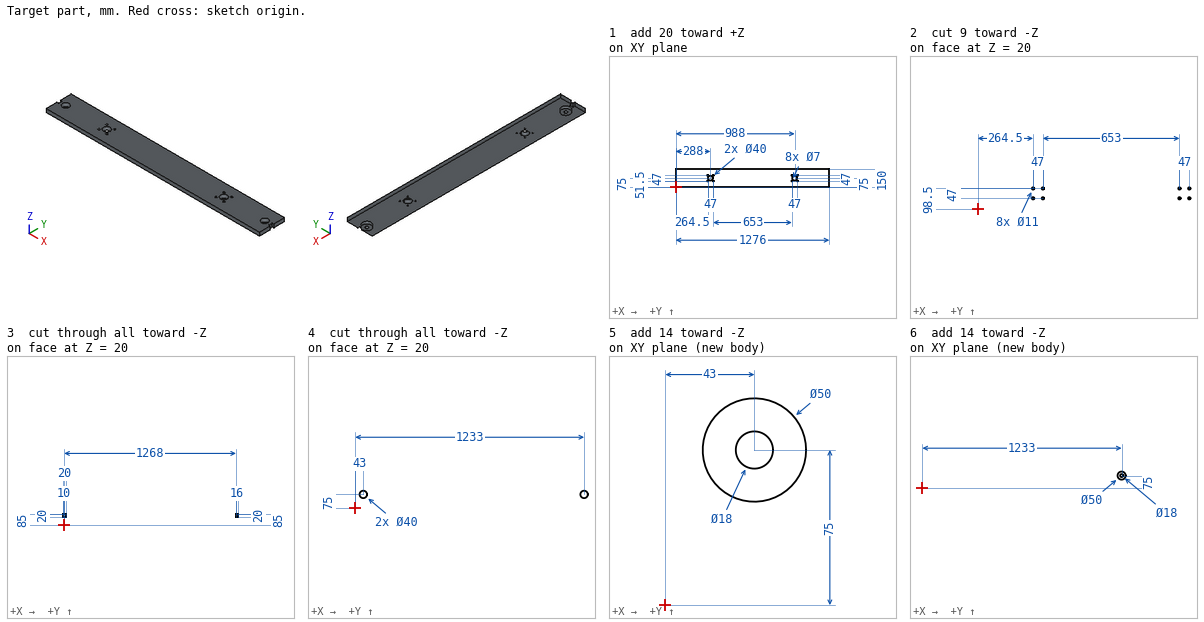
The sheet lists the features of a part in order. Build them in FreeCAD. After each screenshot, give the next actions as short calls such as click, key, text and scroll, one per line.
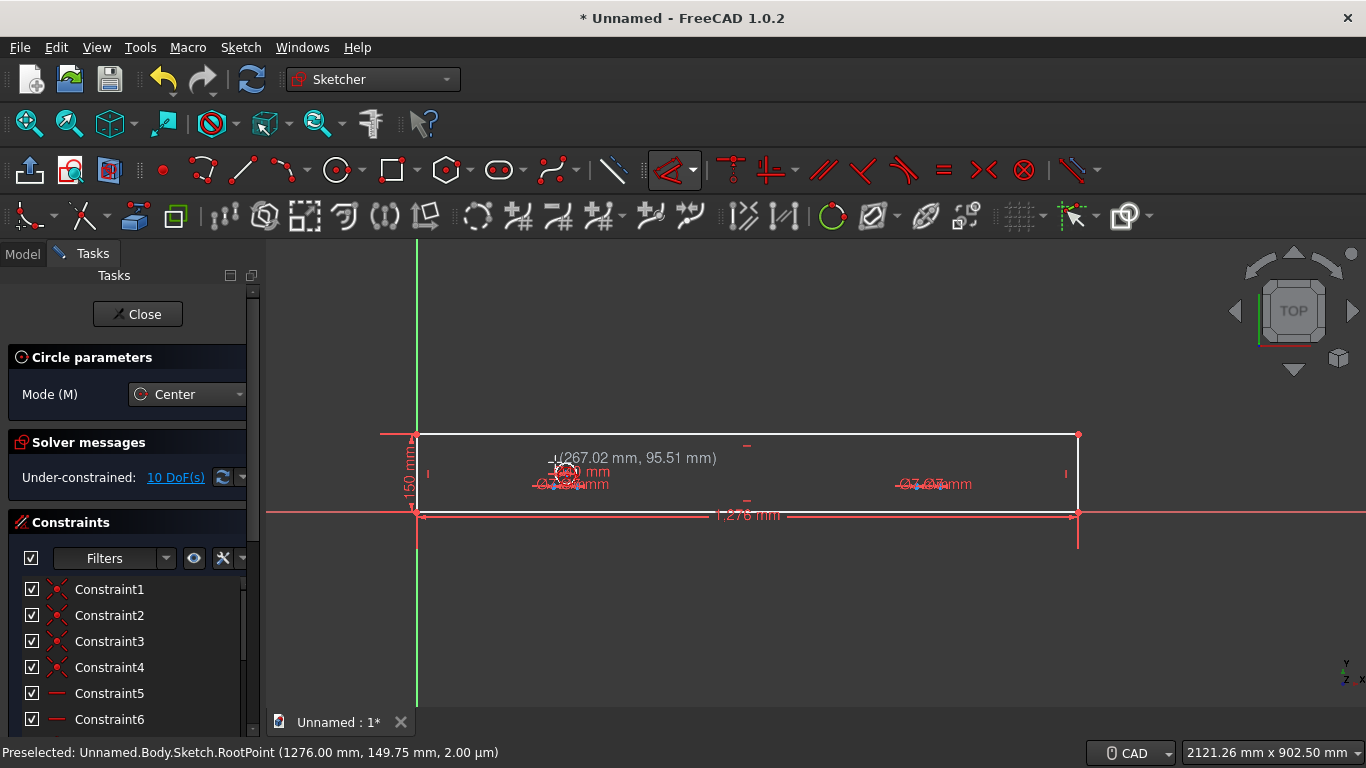
scroll(554, 461, up, 5)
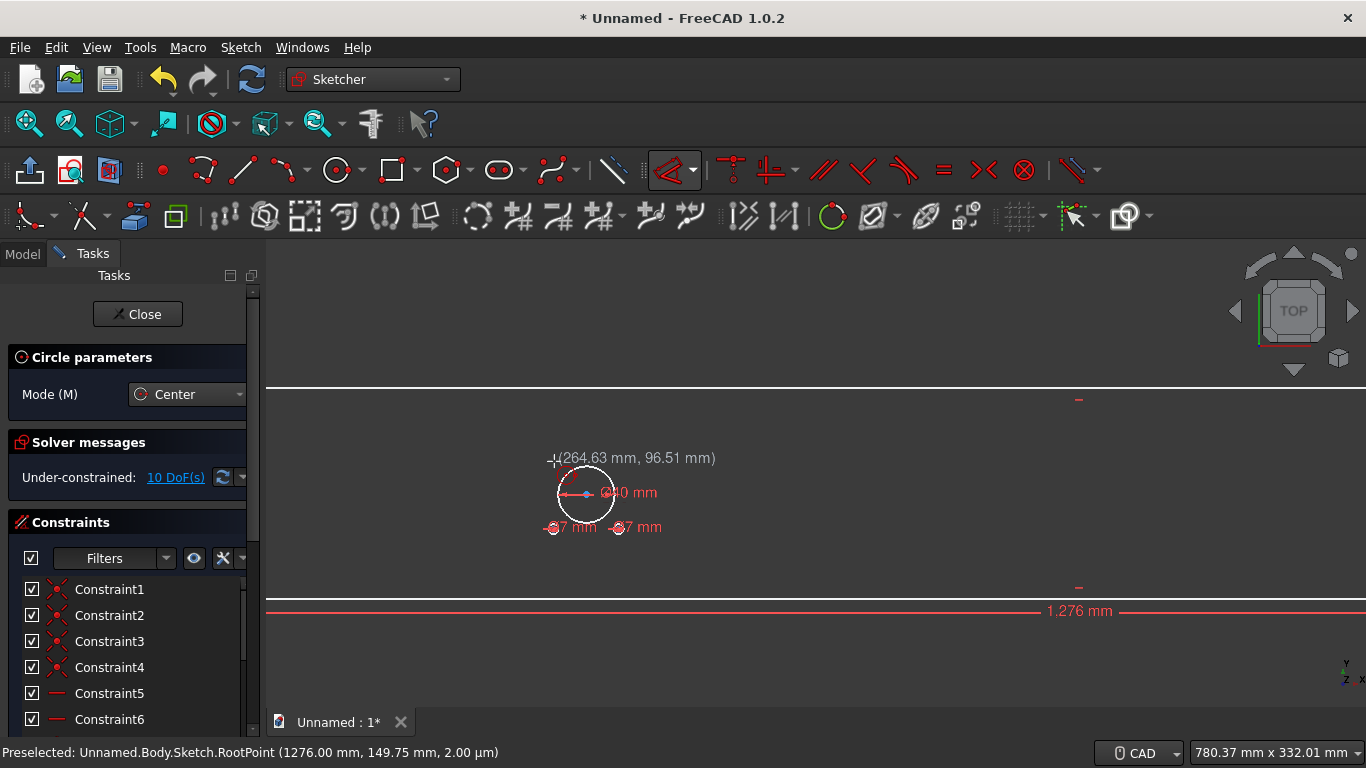
click(553, 460)
move(557, 457)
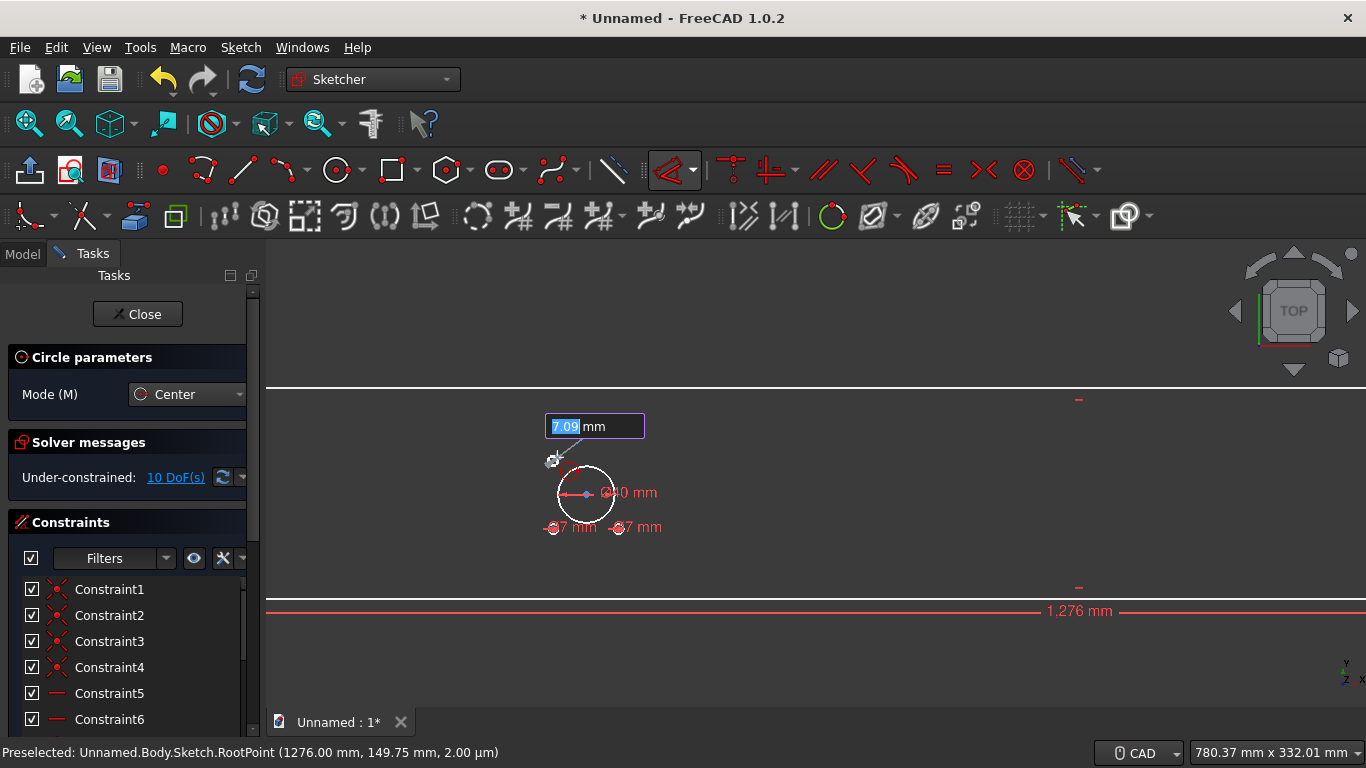
text(7)
key(Return)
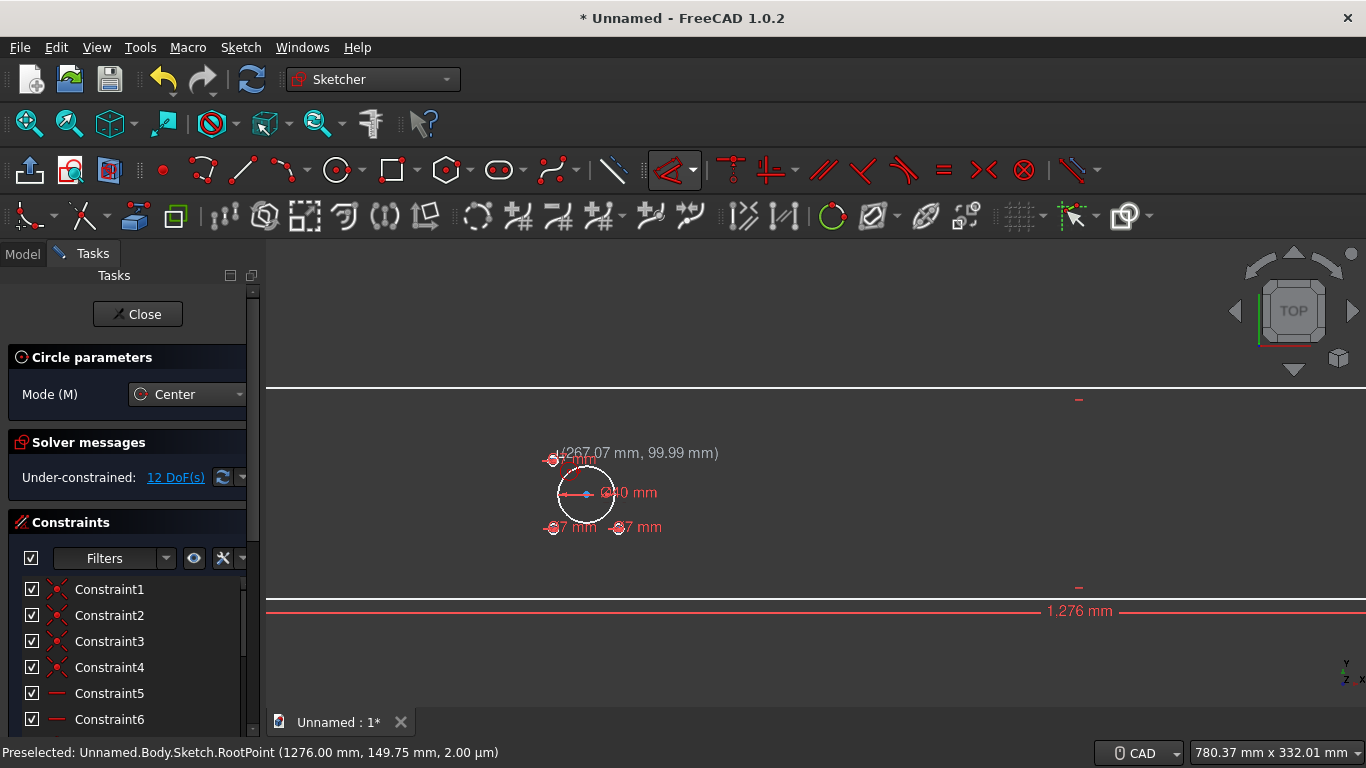
scroll(620, 460, up, 8)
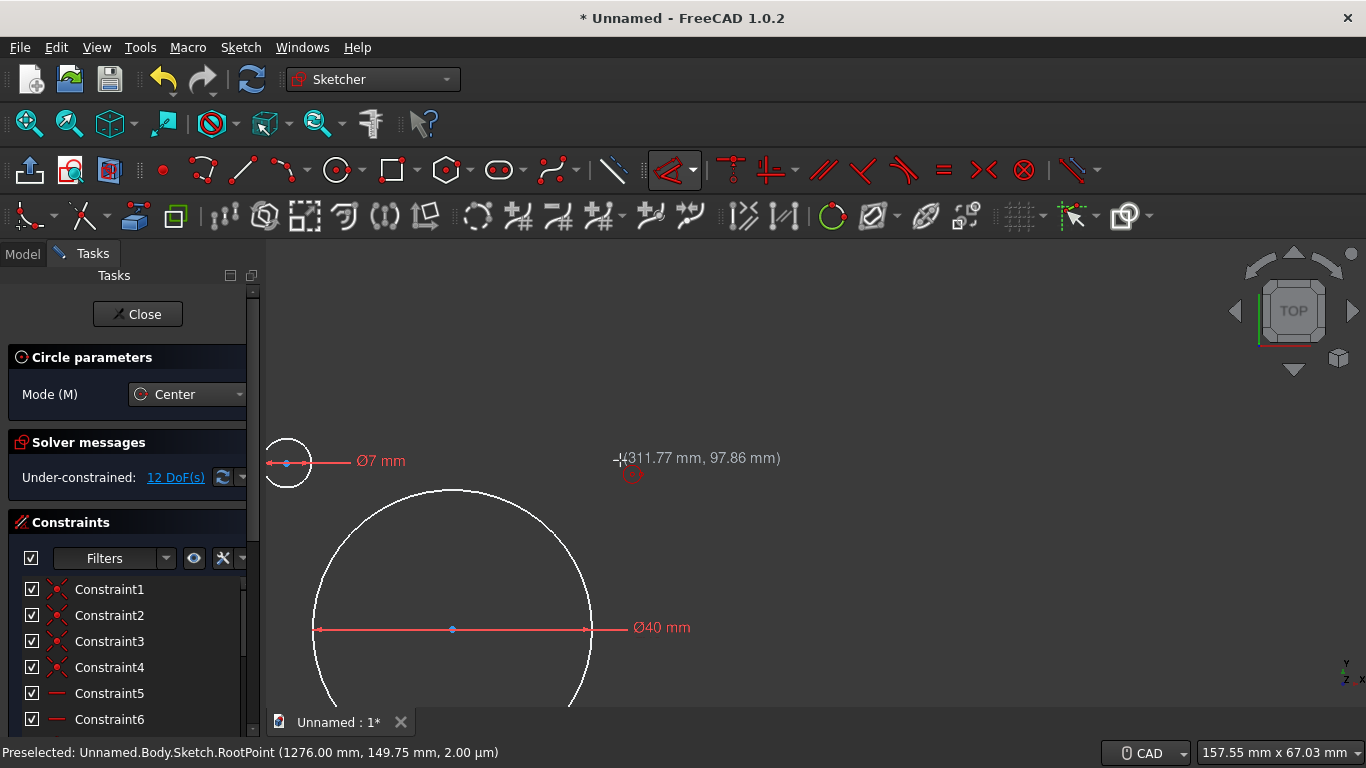
scroll(575, 461, down, 13)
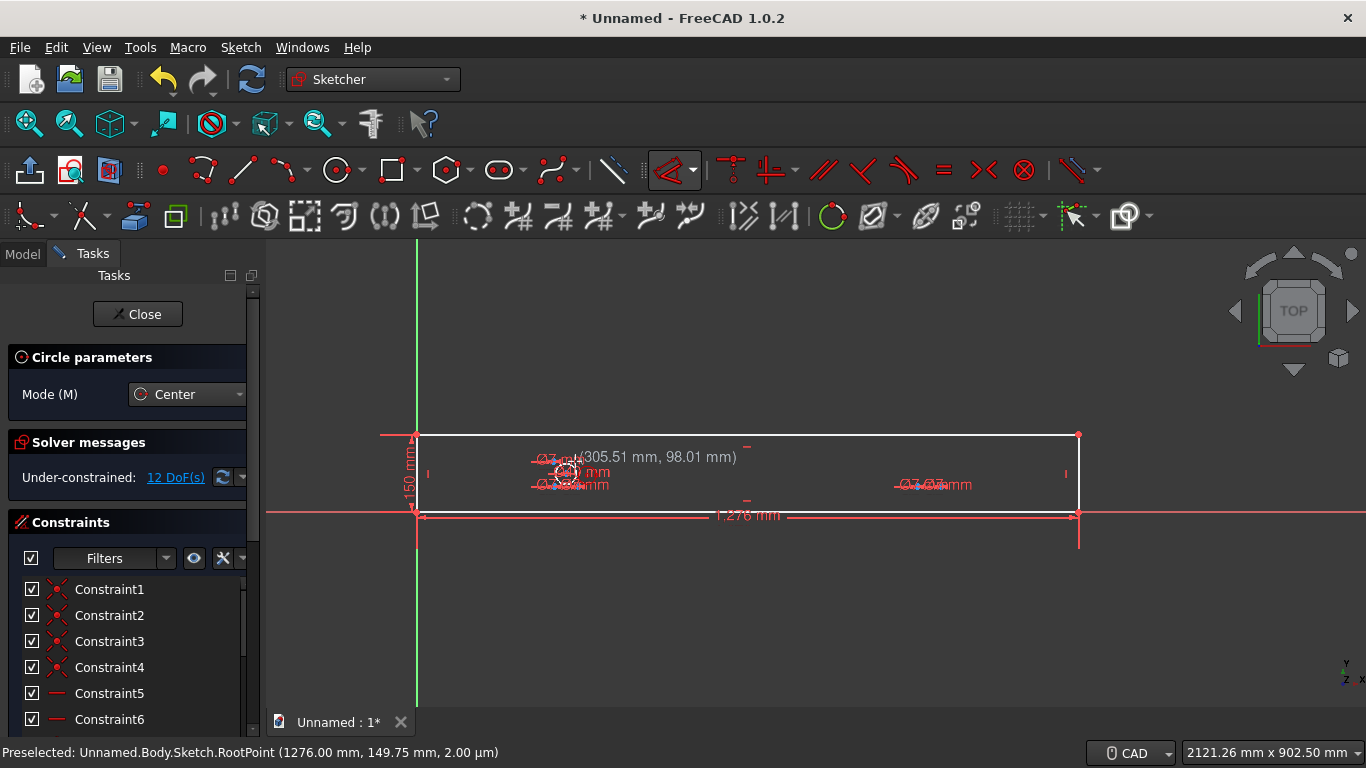
scroll(578, 461, up, 5)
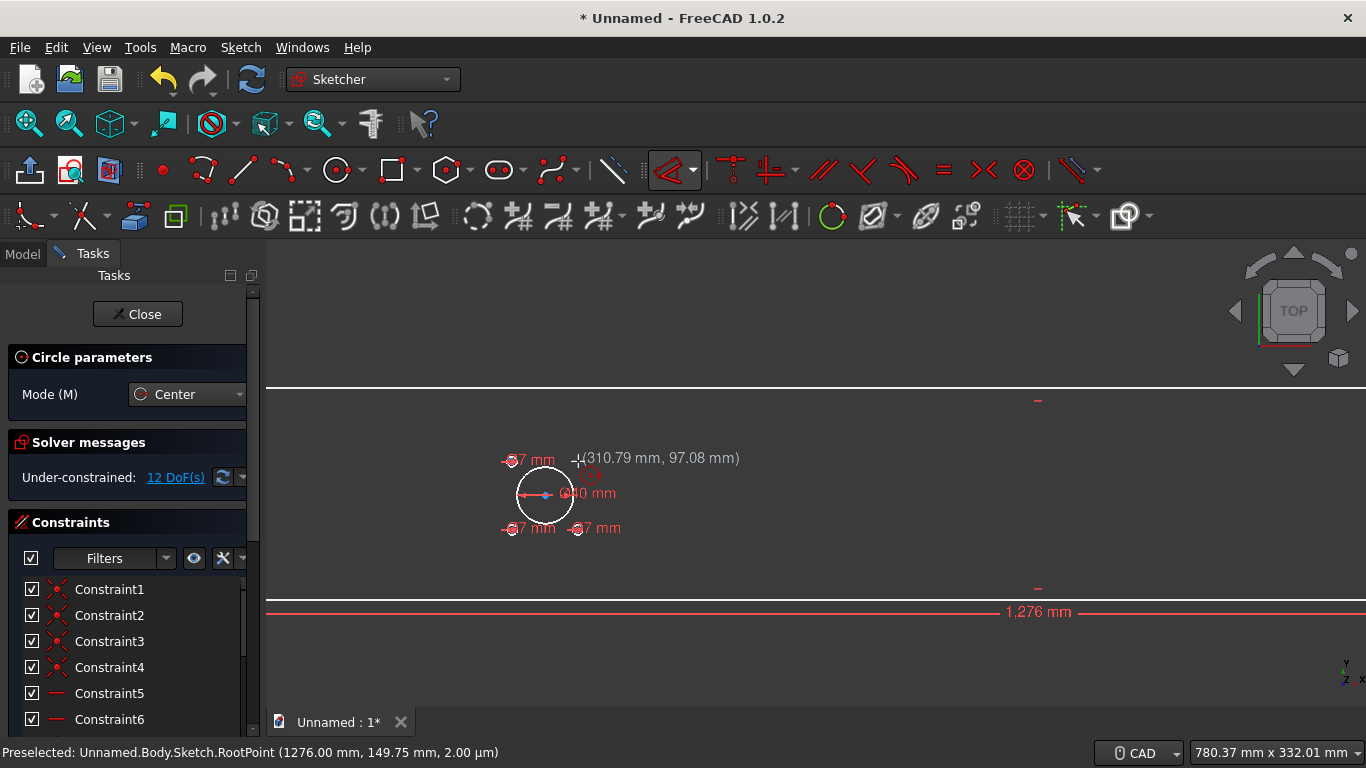
click(579, 461)
move(582, 457)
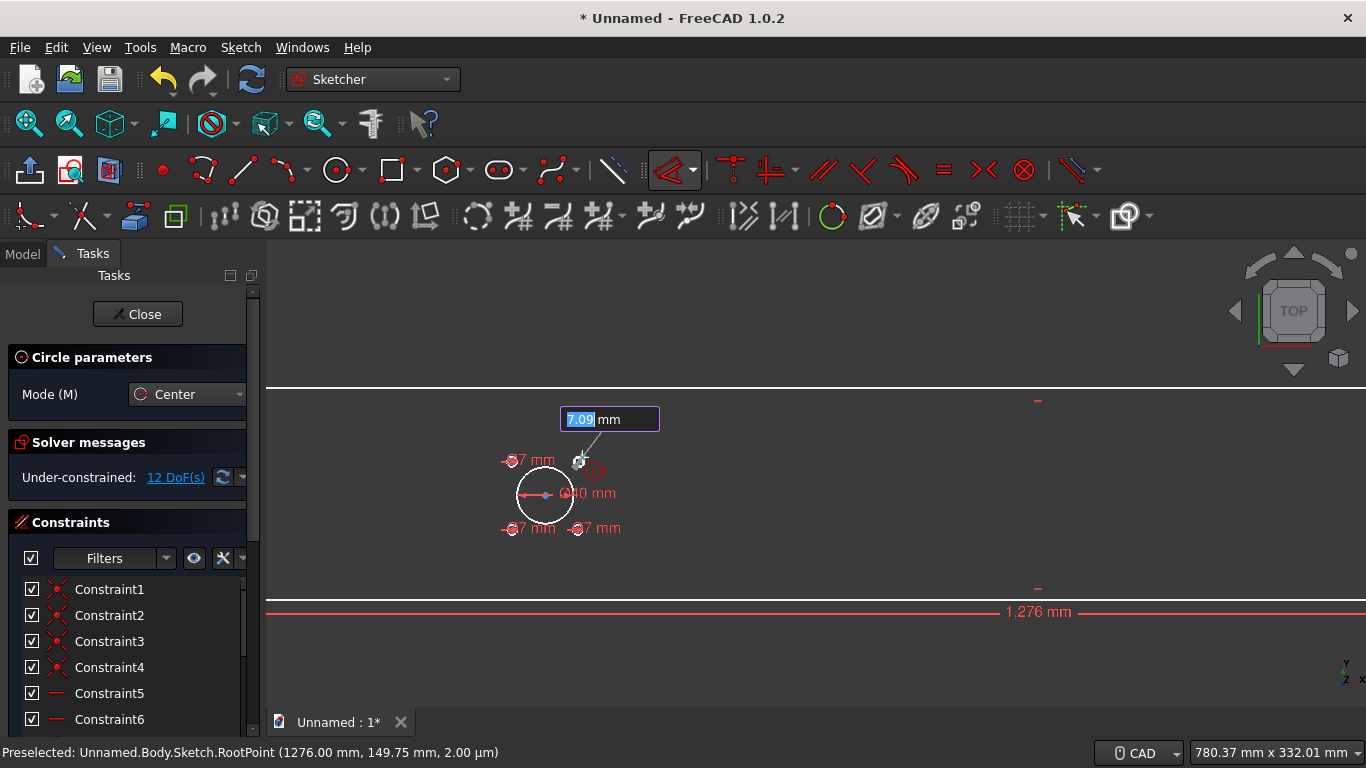
text(7)
key(Return)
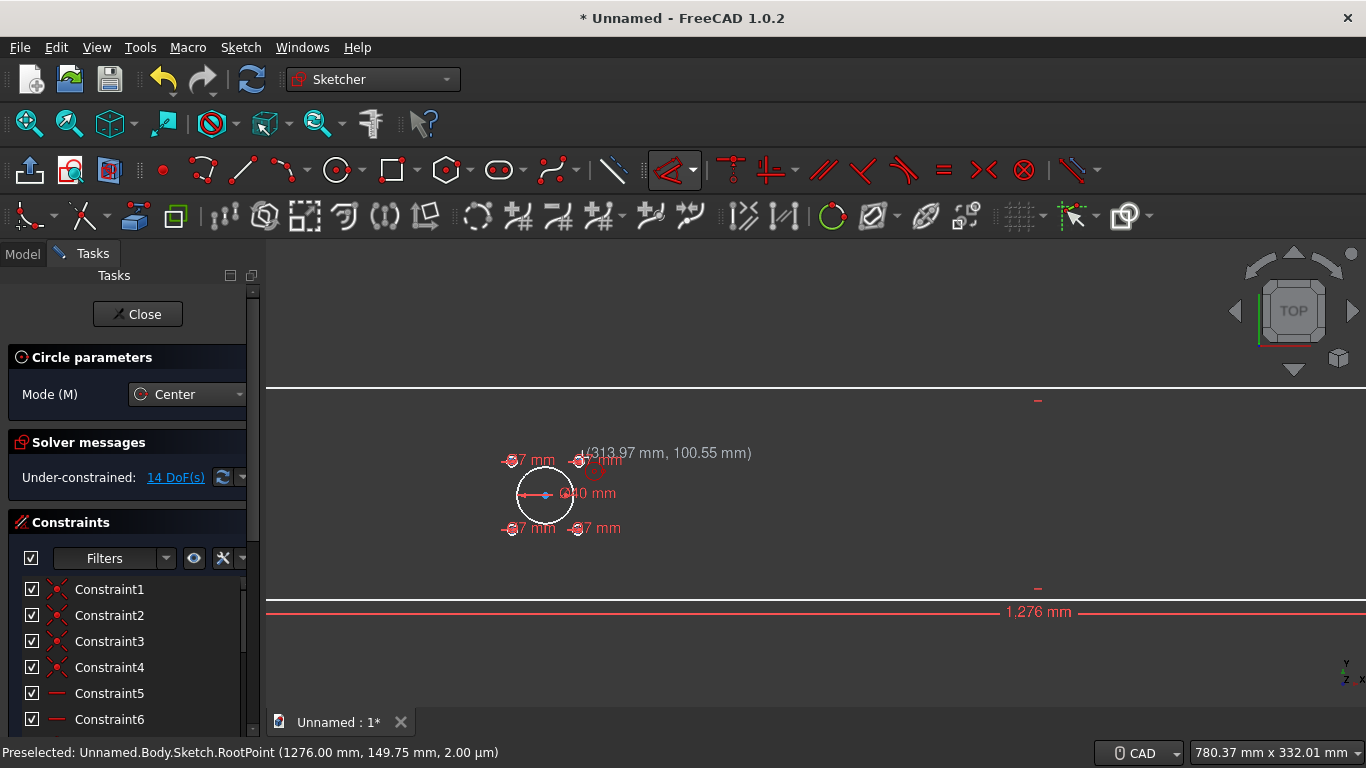
scroll(578, 461, down, 5)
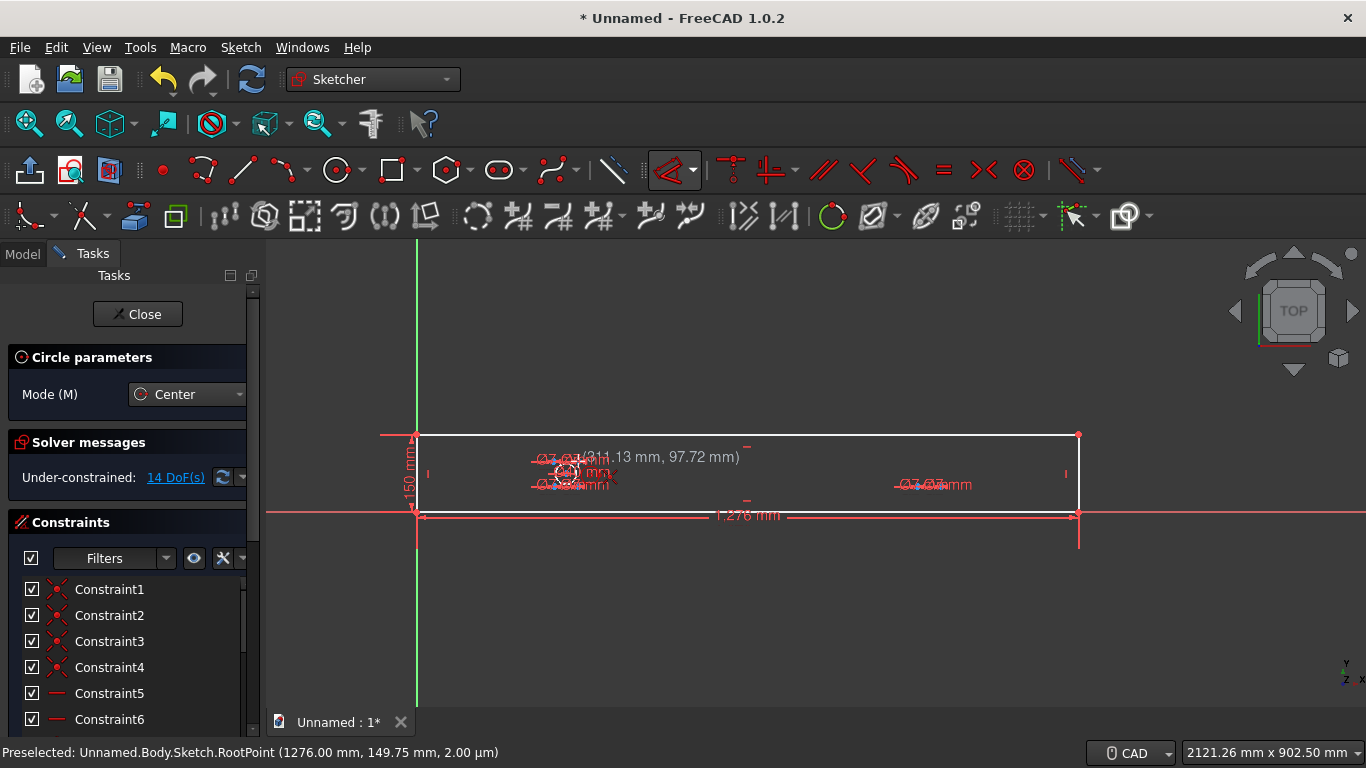
scroll(929, 473, up, 4)